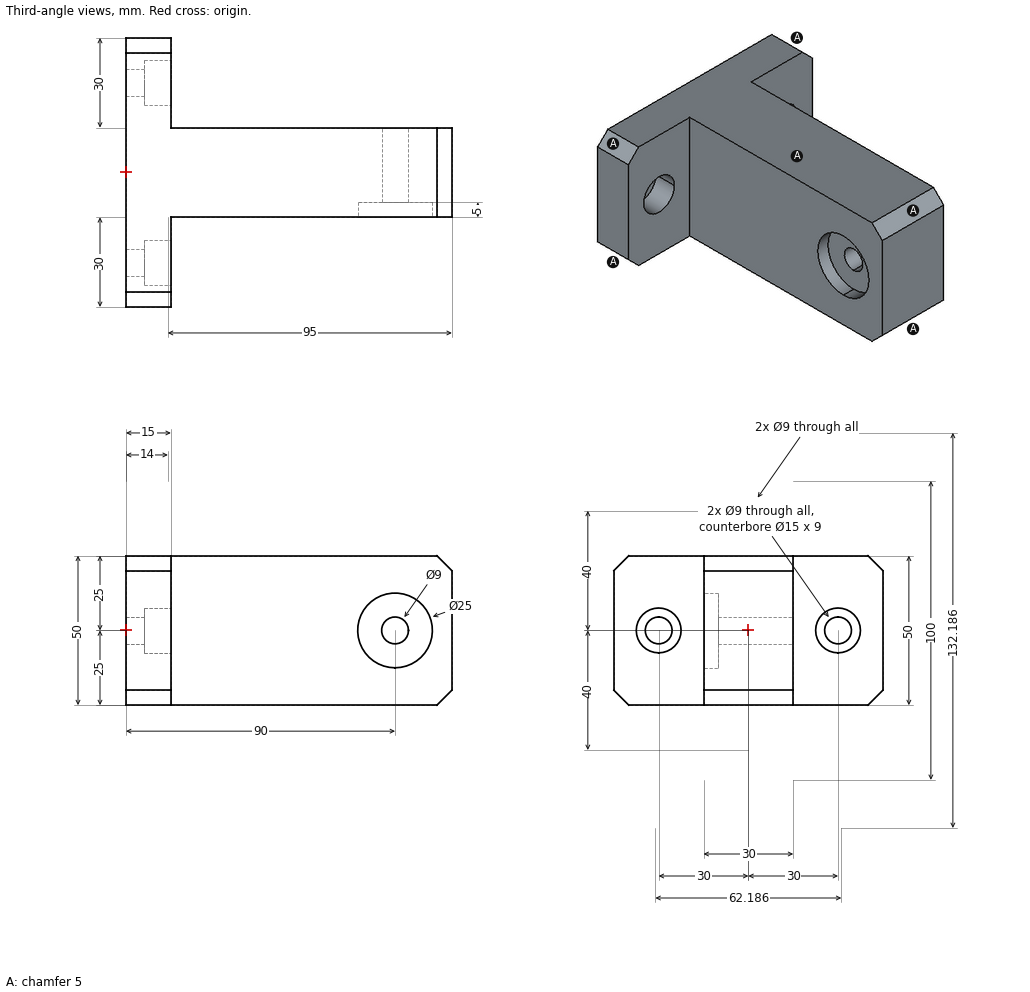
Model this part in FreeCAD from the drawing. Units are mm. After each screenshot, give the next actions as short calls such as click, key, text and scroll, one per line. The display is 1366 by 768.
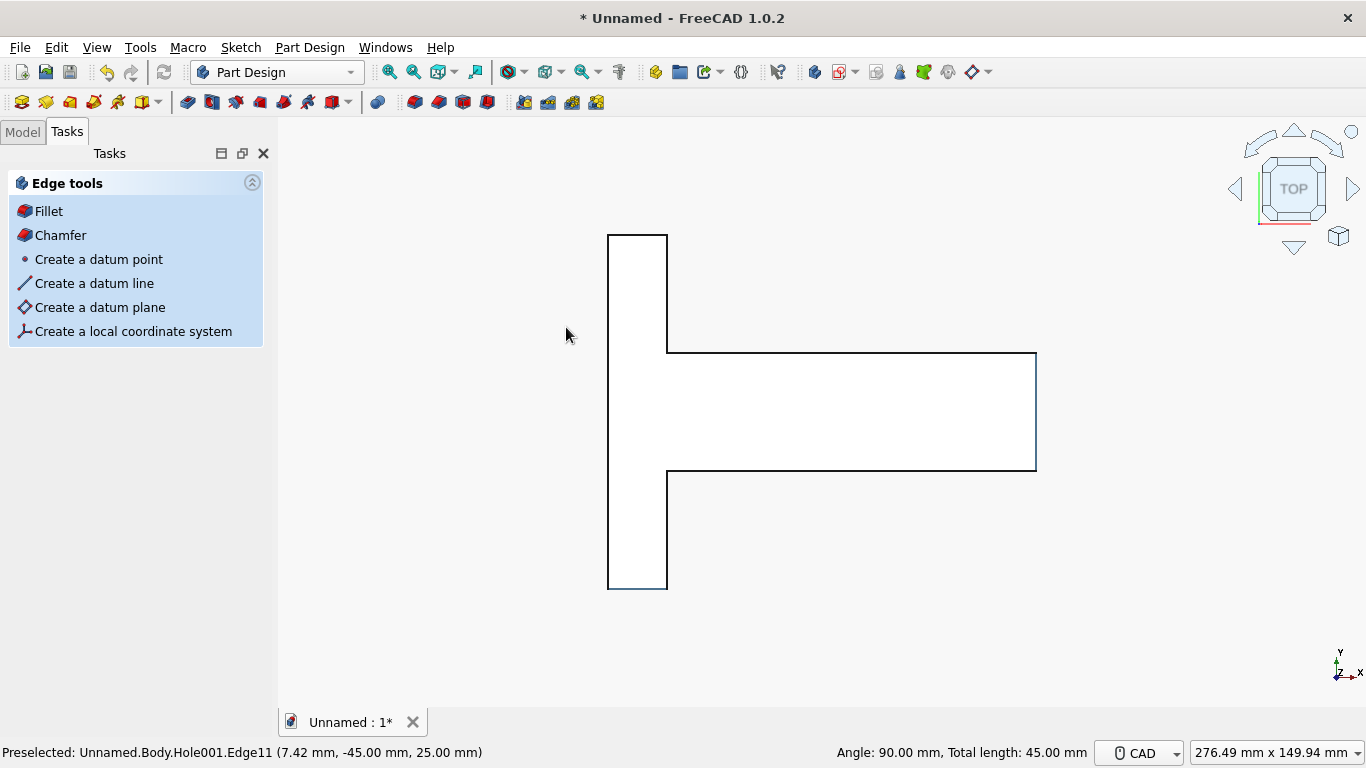
click(637, 234, ctrl)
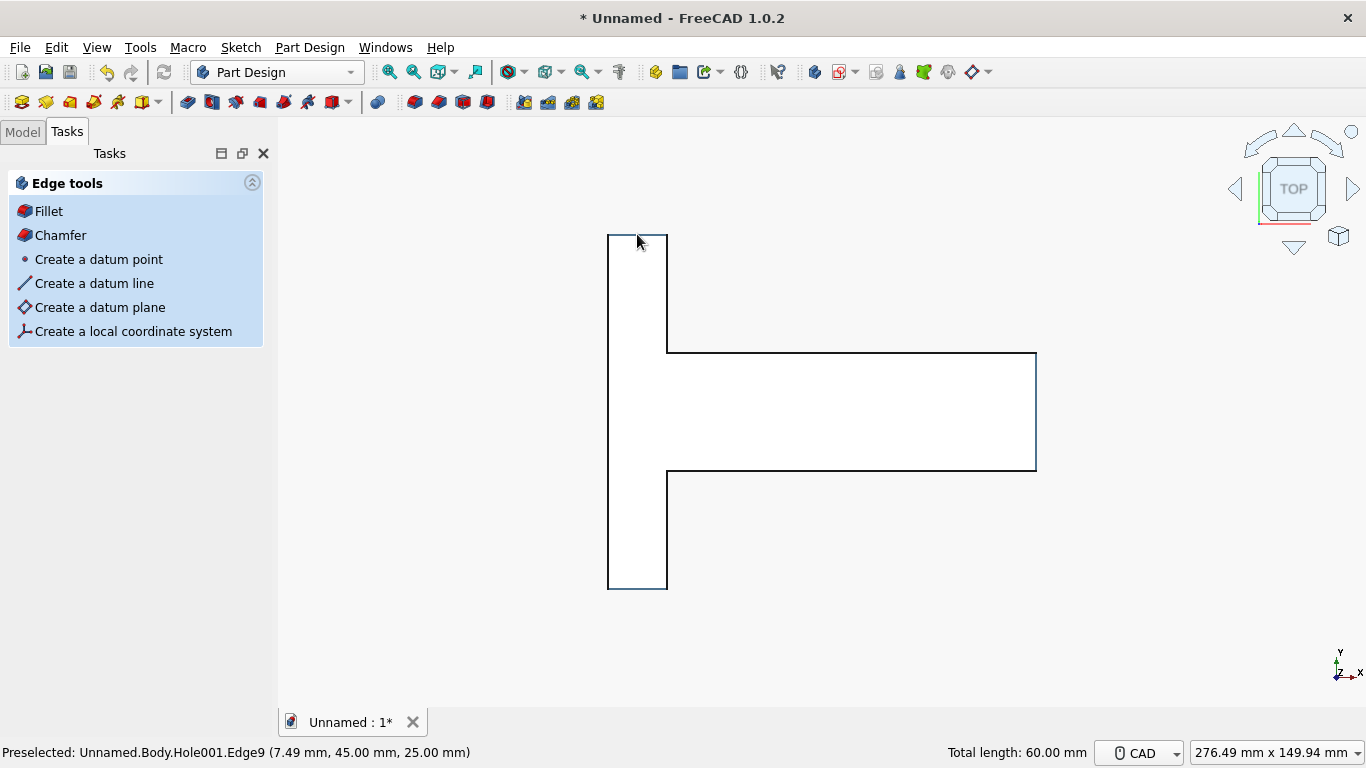
key(0)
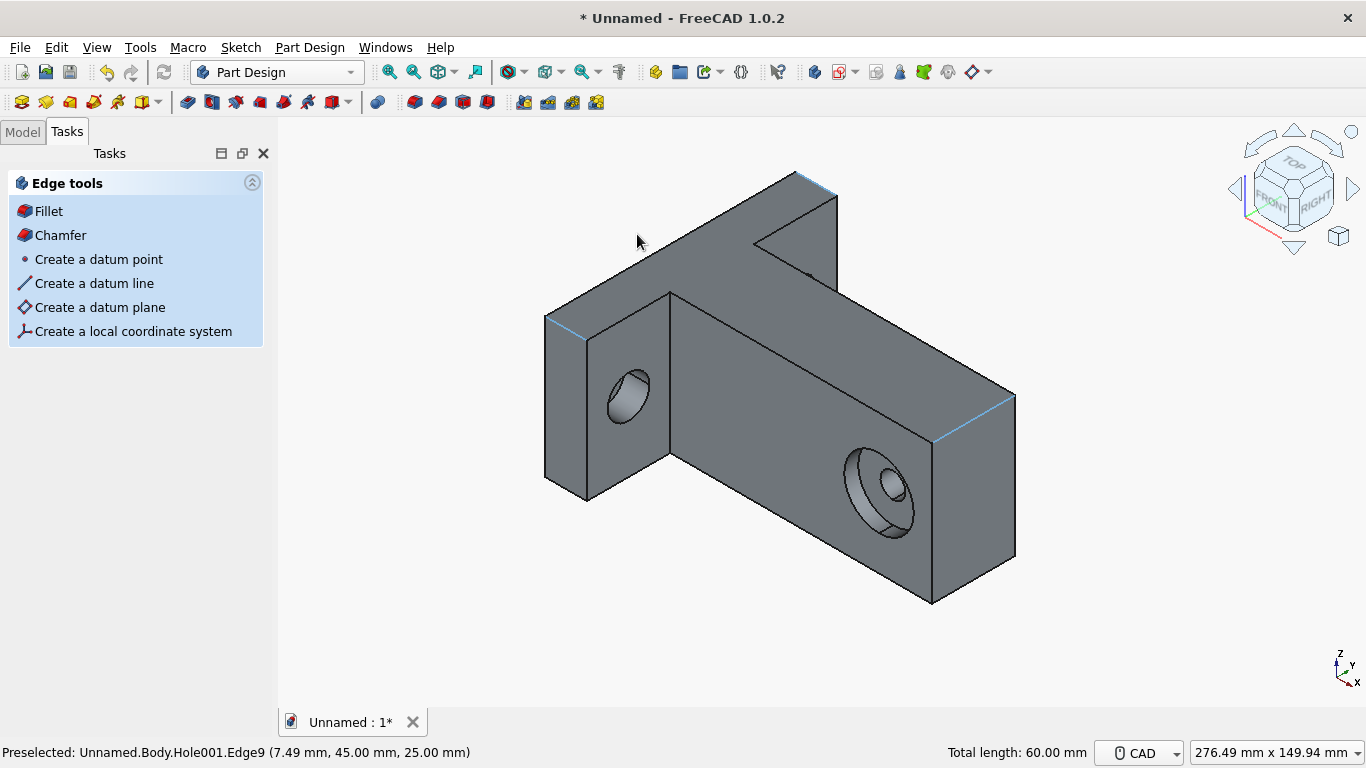
key(1)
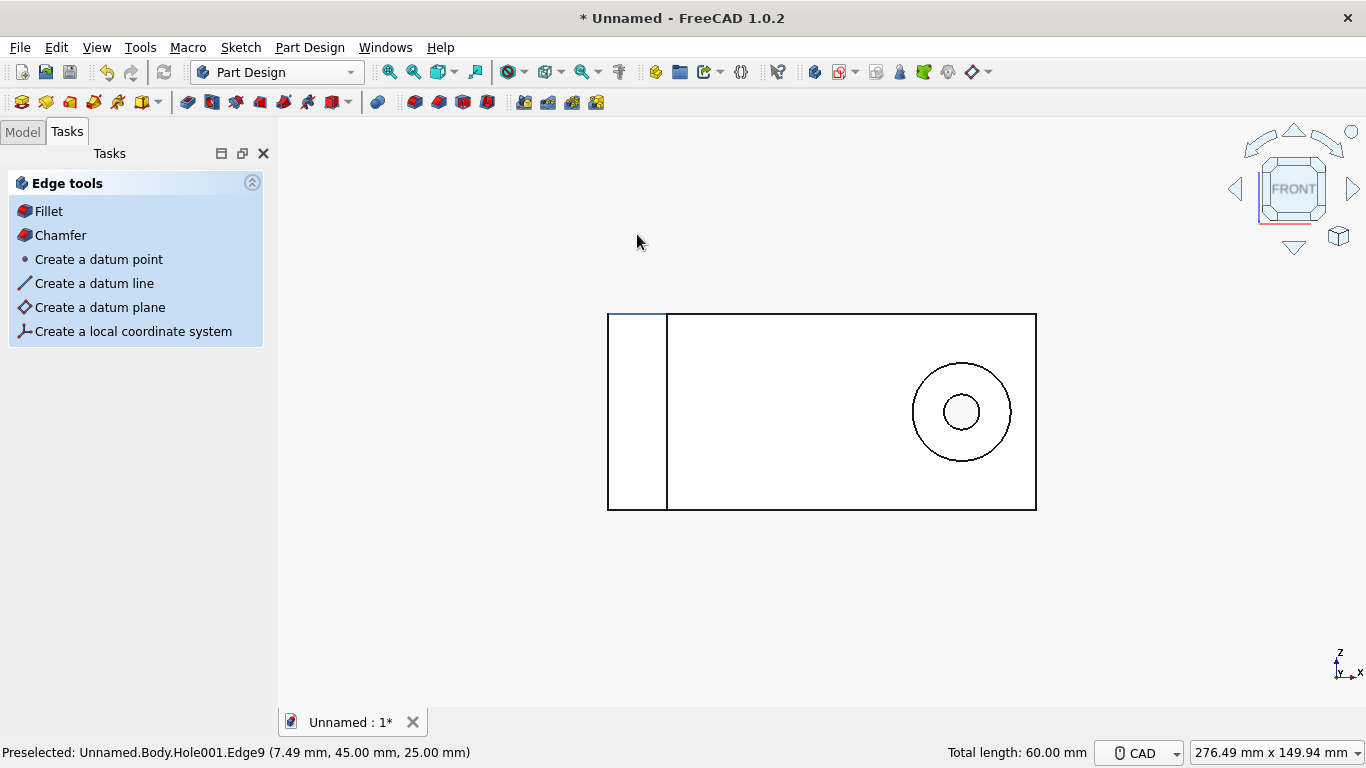
click(390, 72)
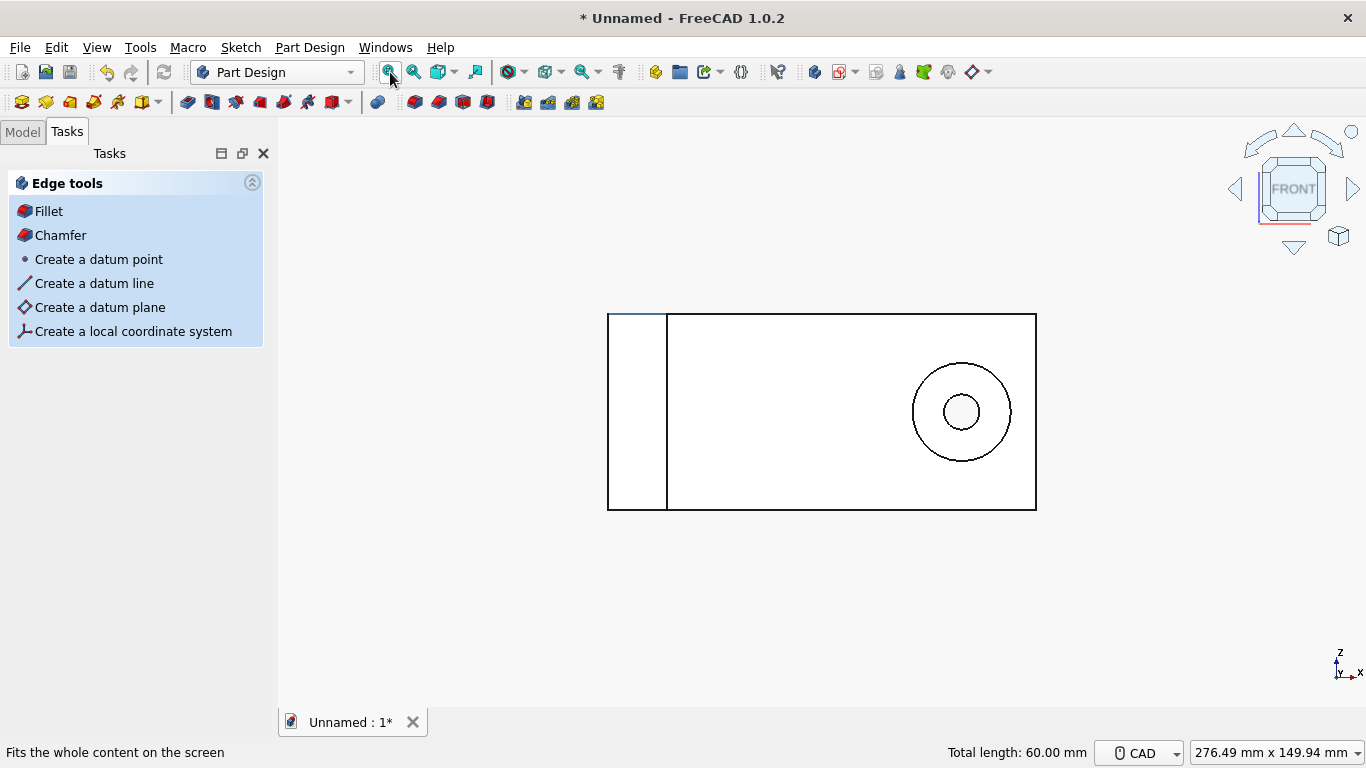
click(637, 509, ctrl)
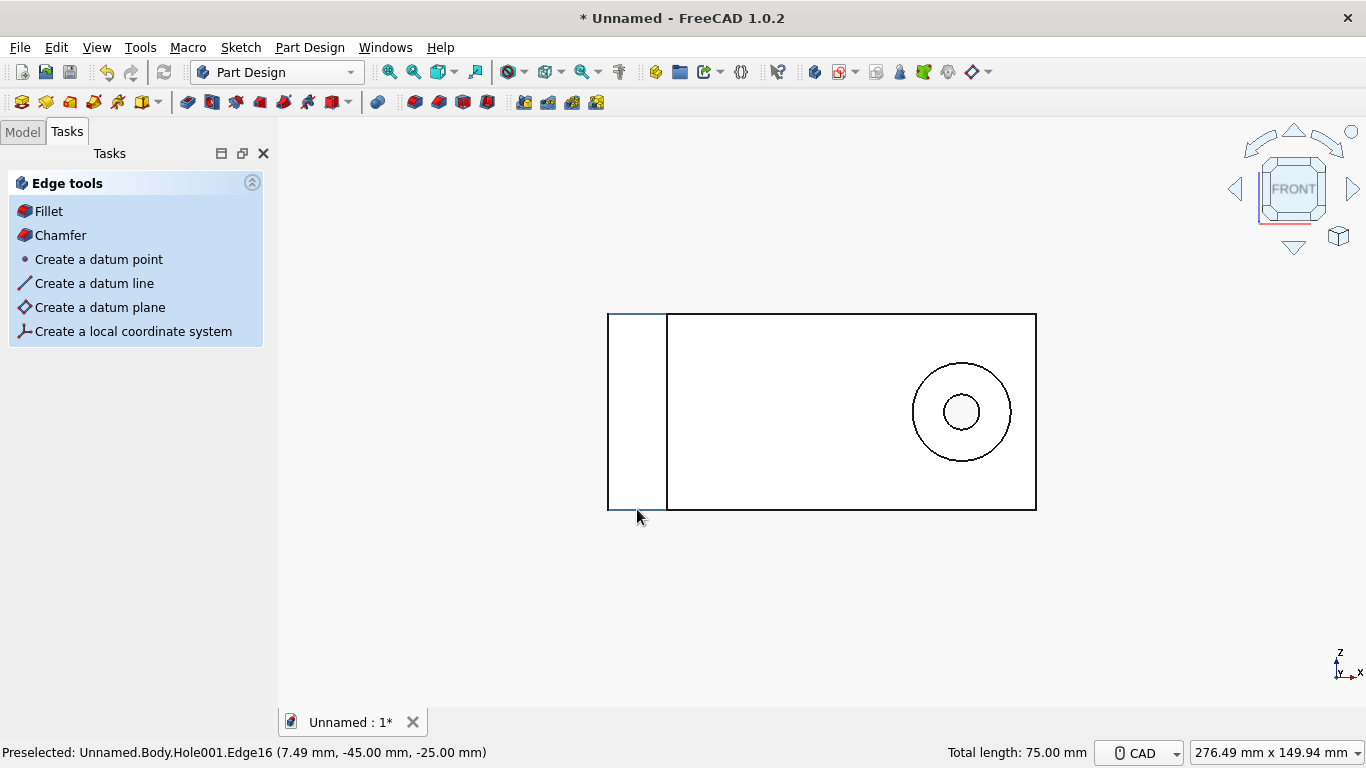
key(3)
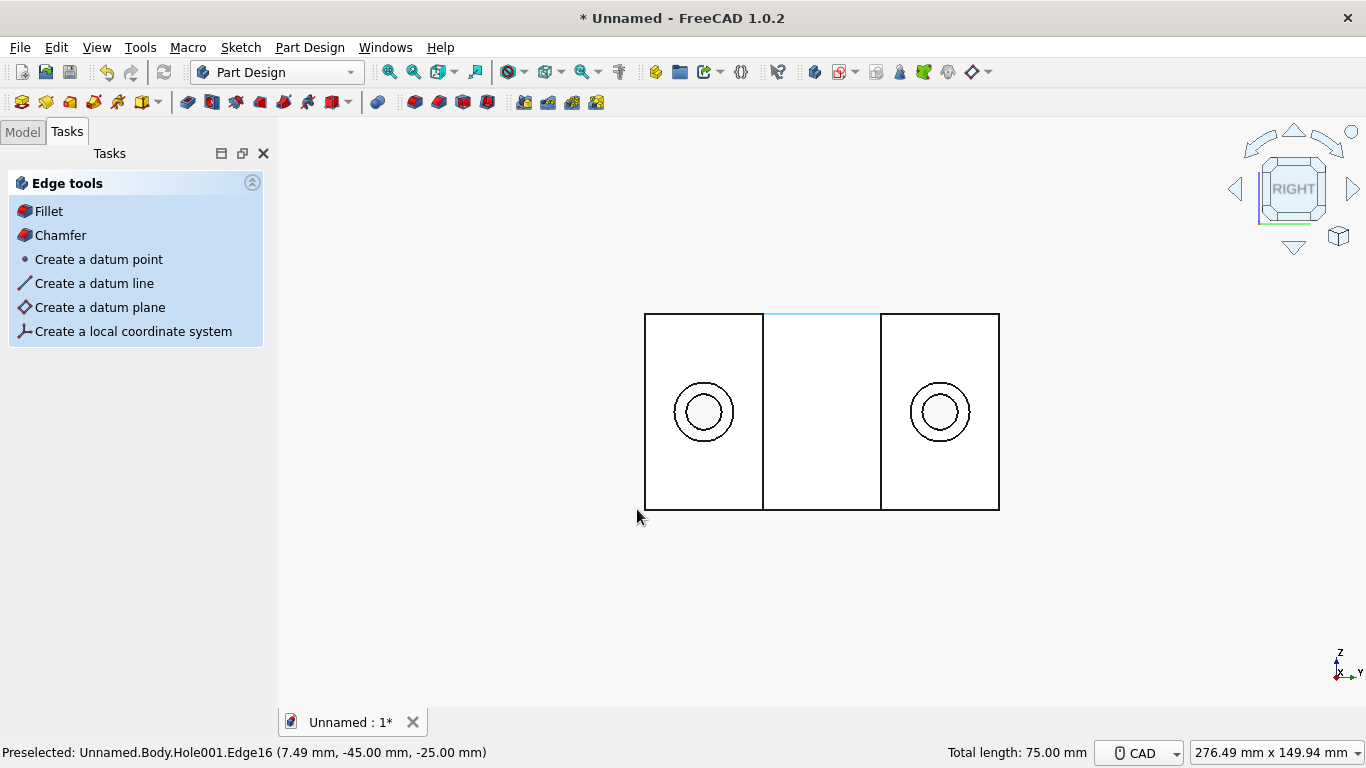
click(390, 72)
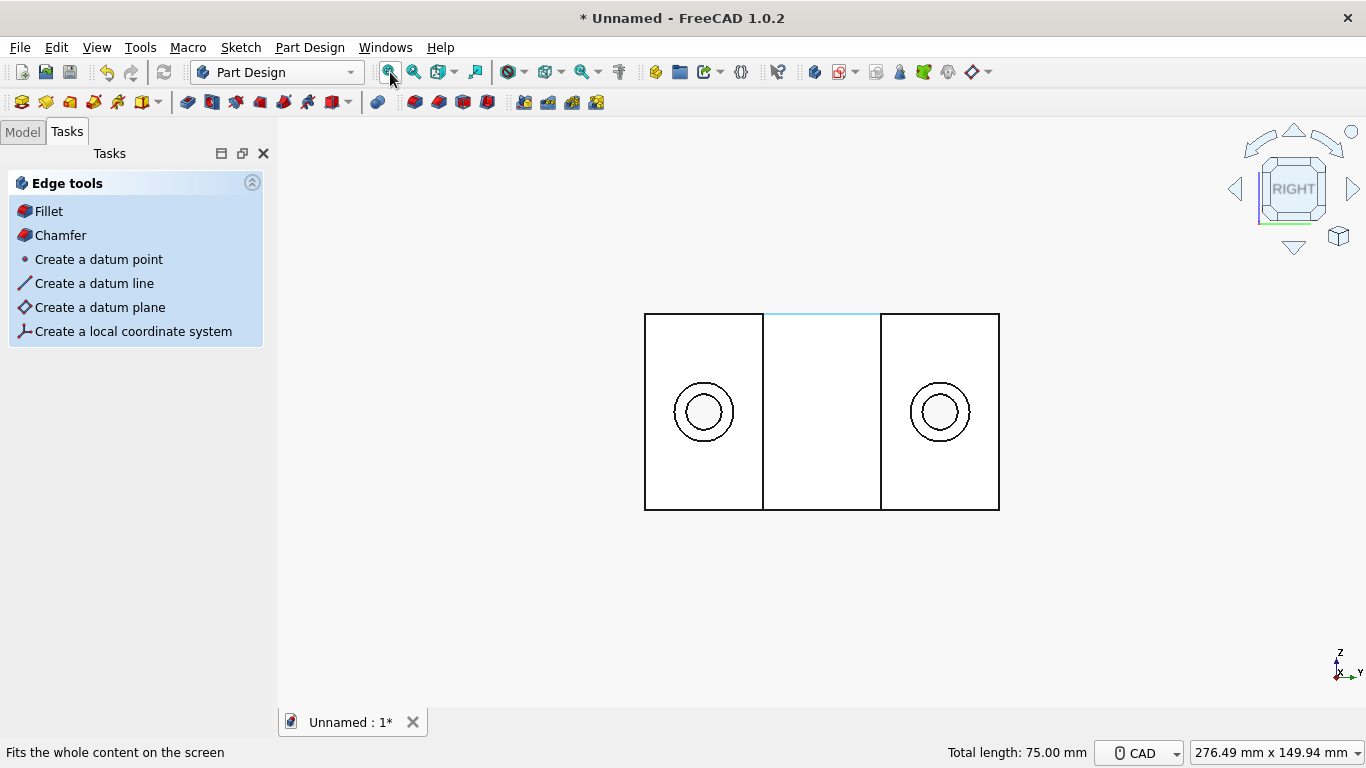
click(822, 509, ctrl)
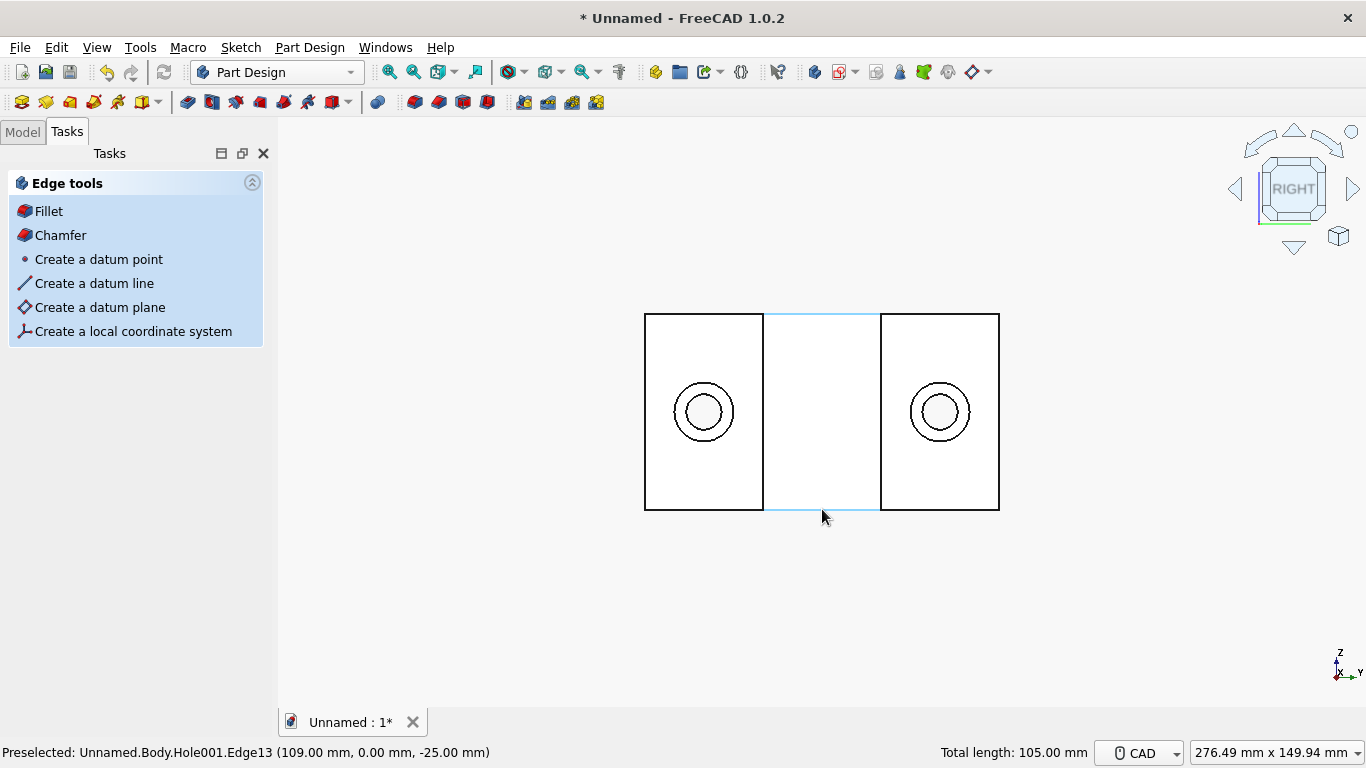
key(5)